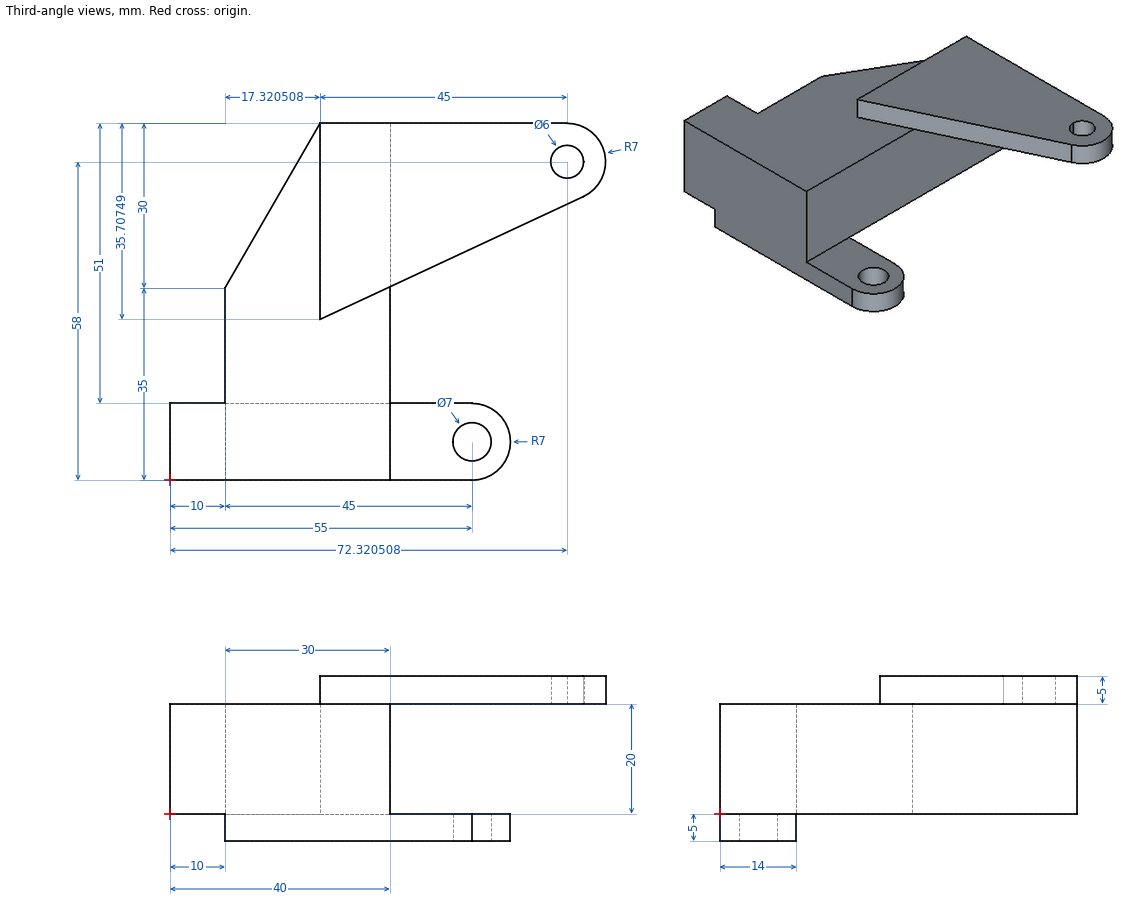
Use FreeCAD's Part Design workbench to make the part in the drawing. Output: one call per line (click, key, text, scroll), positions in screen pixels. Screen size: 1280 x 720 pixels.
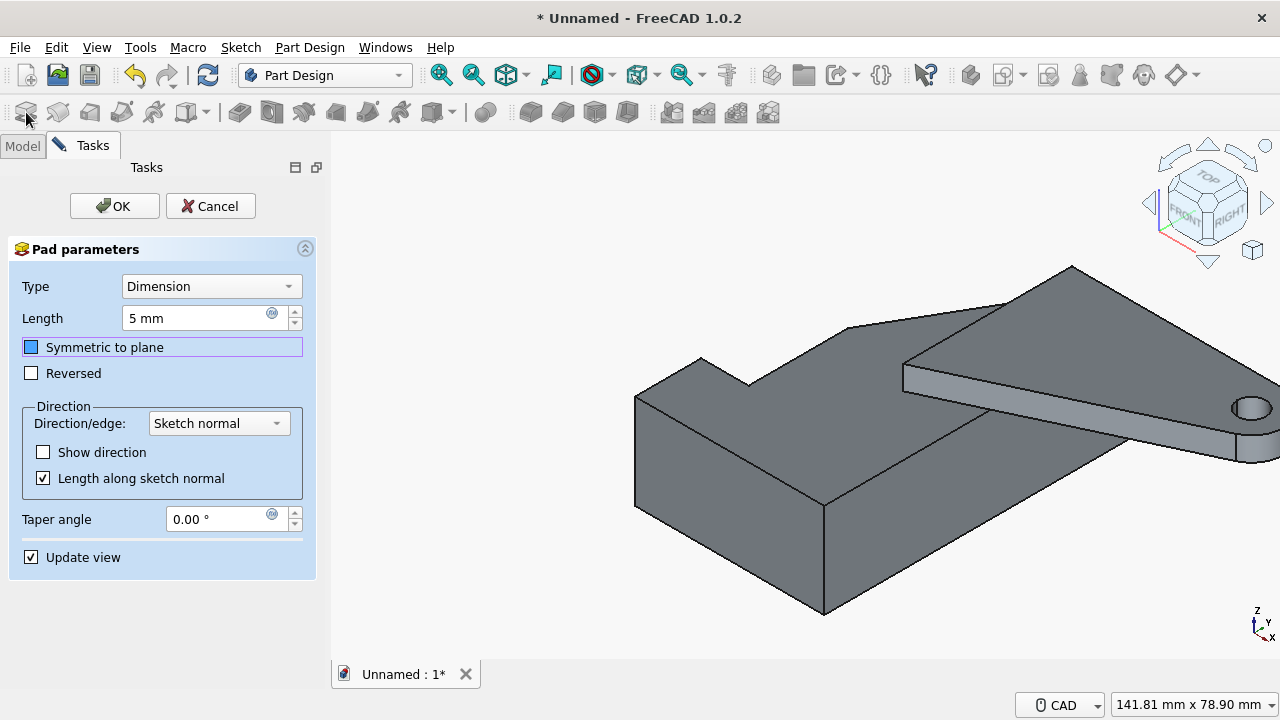
click(115, 206)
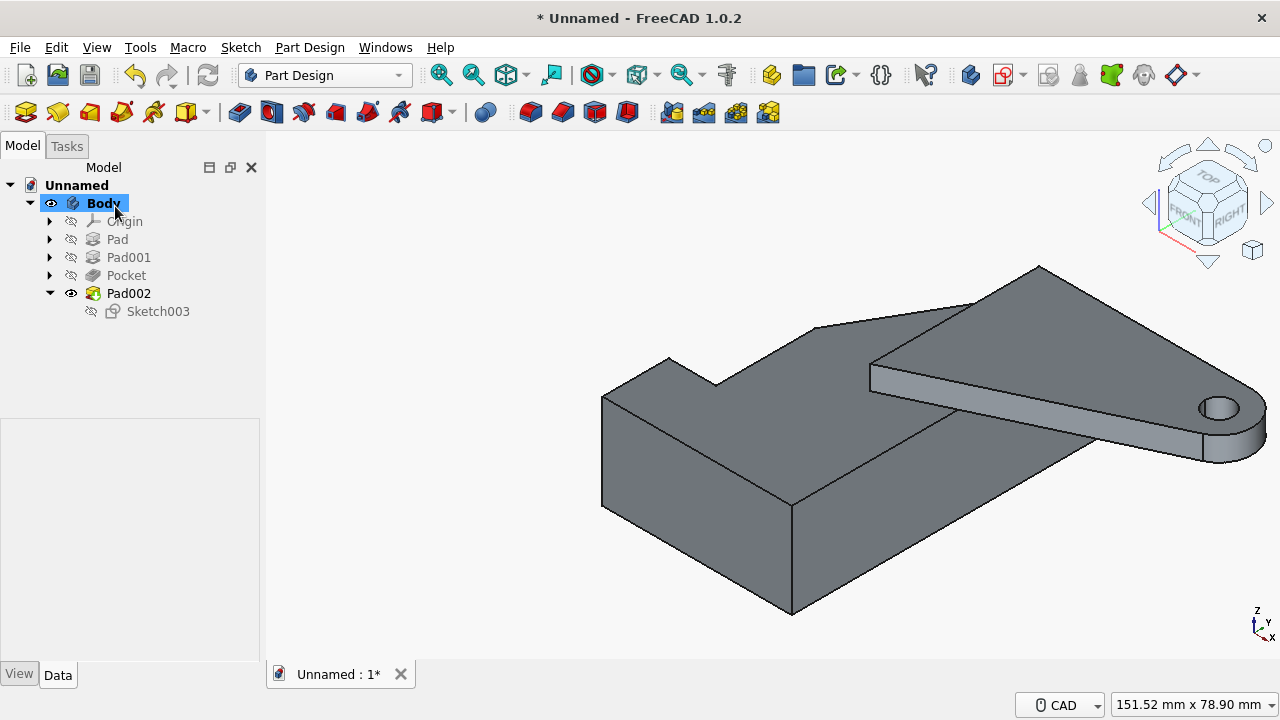
click(442, 76)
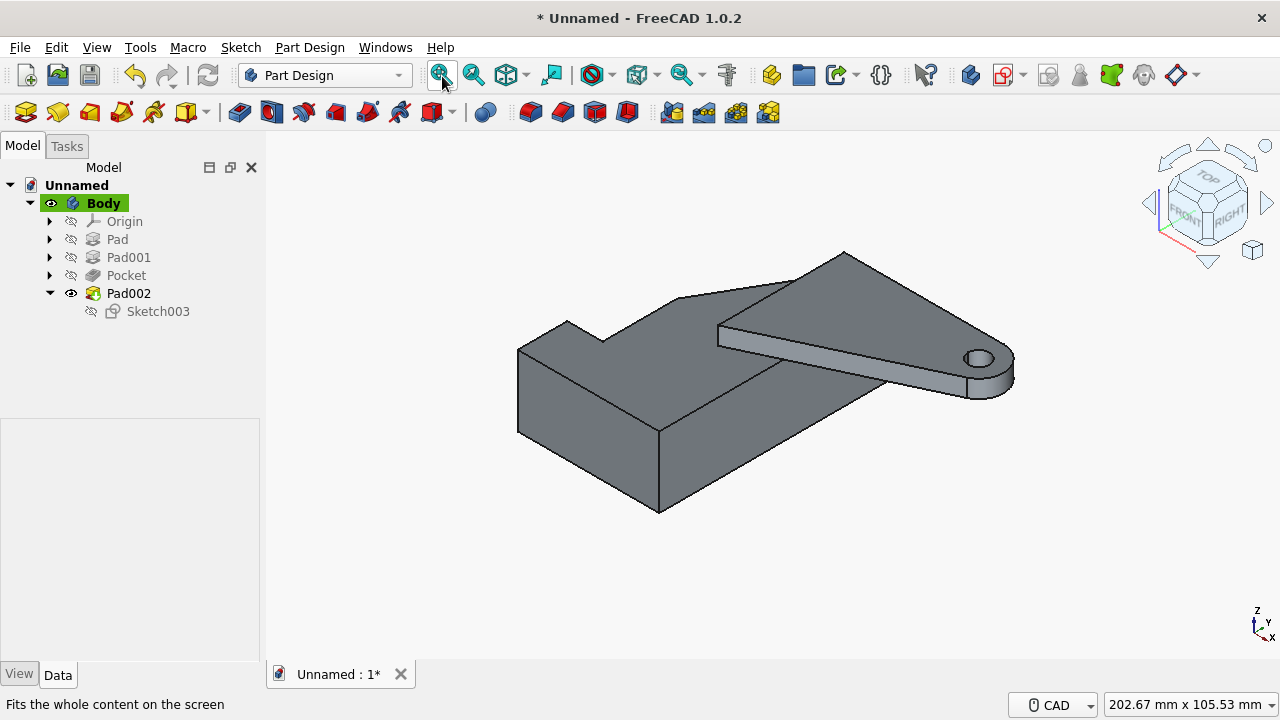
click(1004, 76)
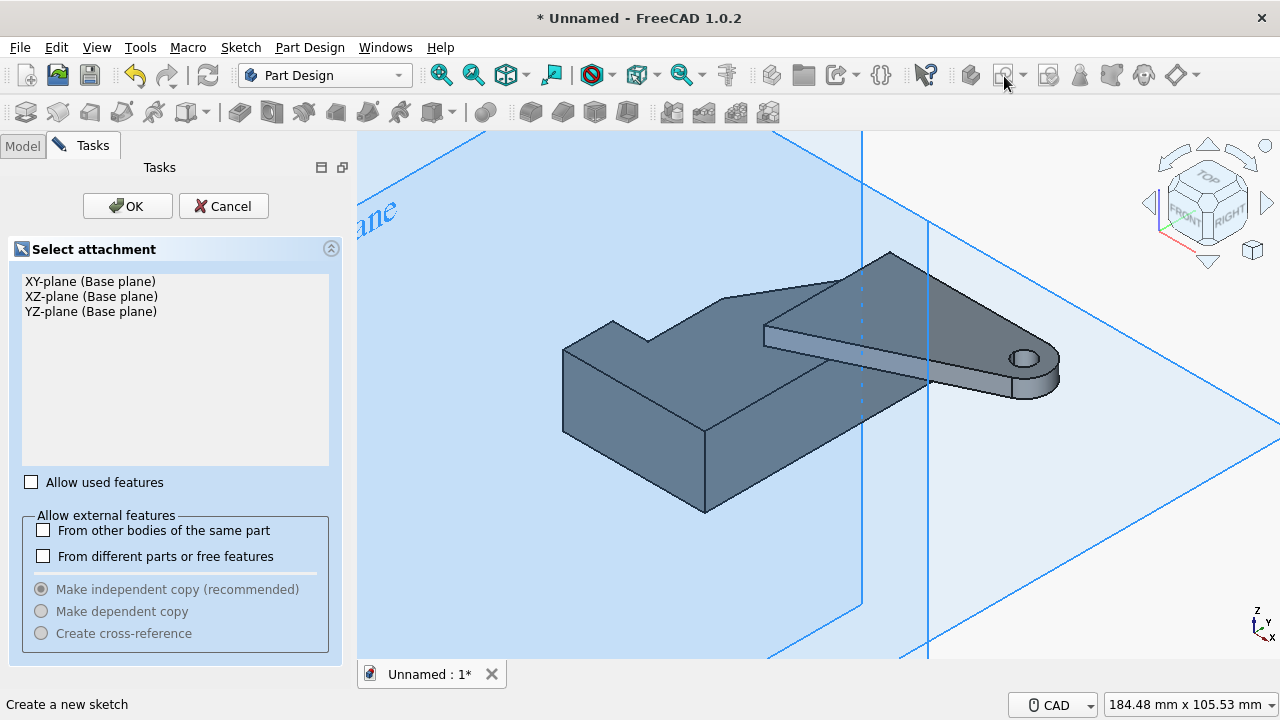
click(82, 282)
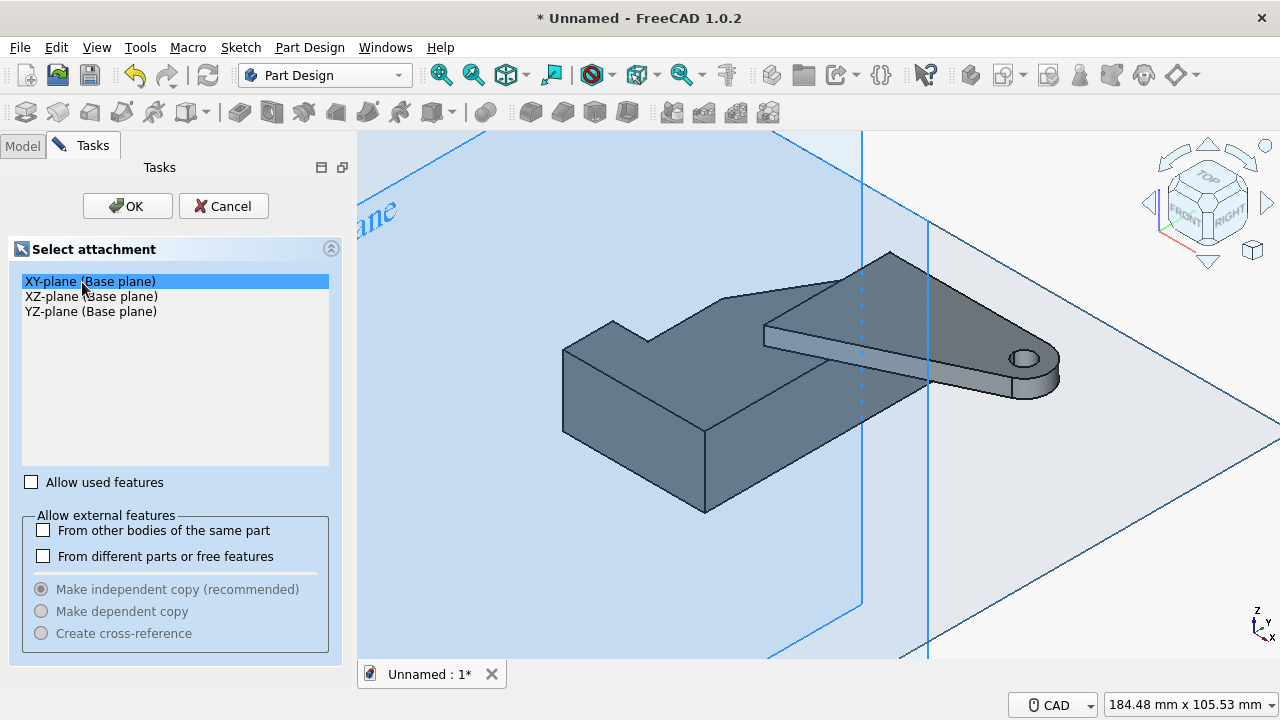
click(128, 206)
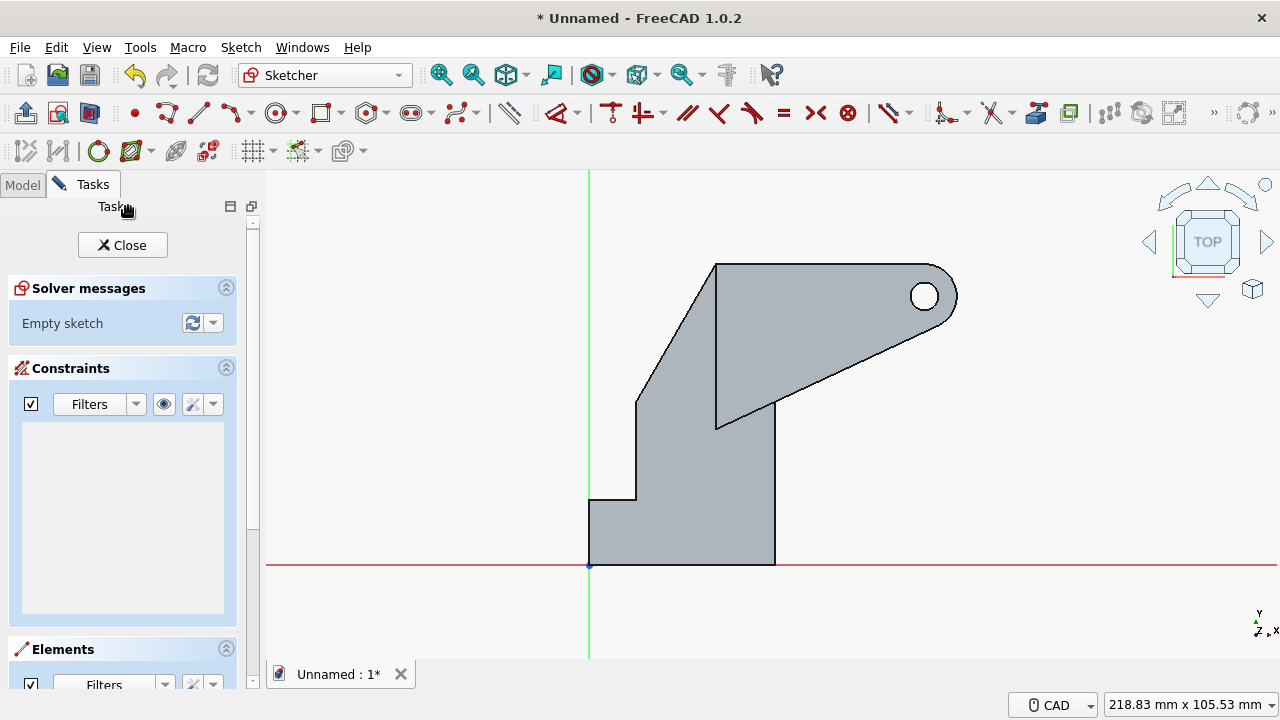
click(90, 114)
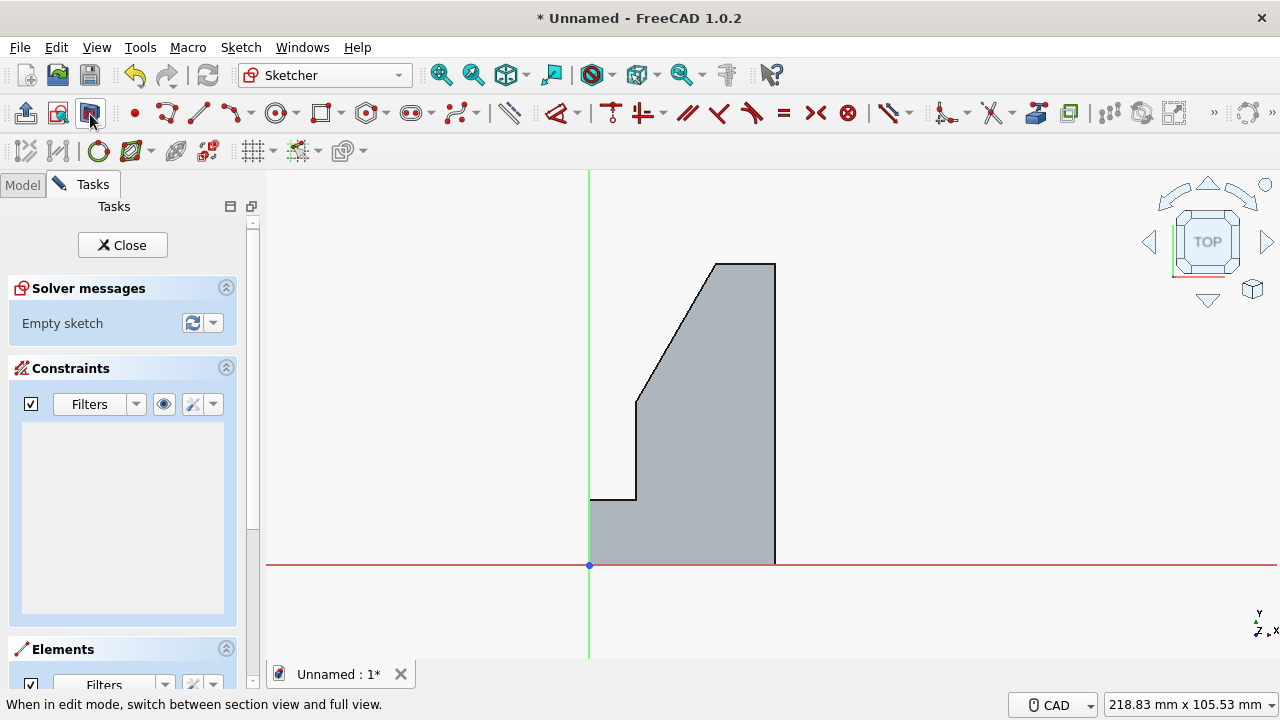
scroll(756, 629, up, 4)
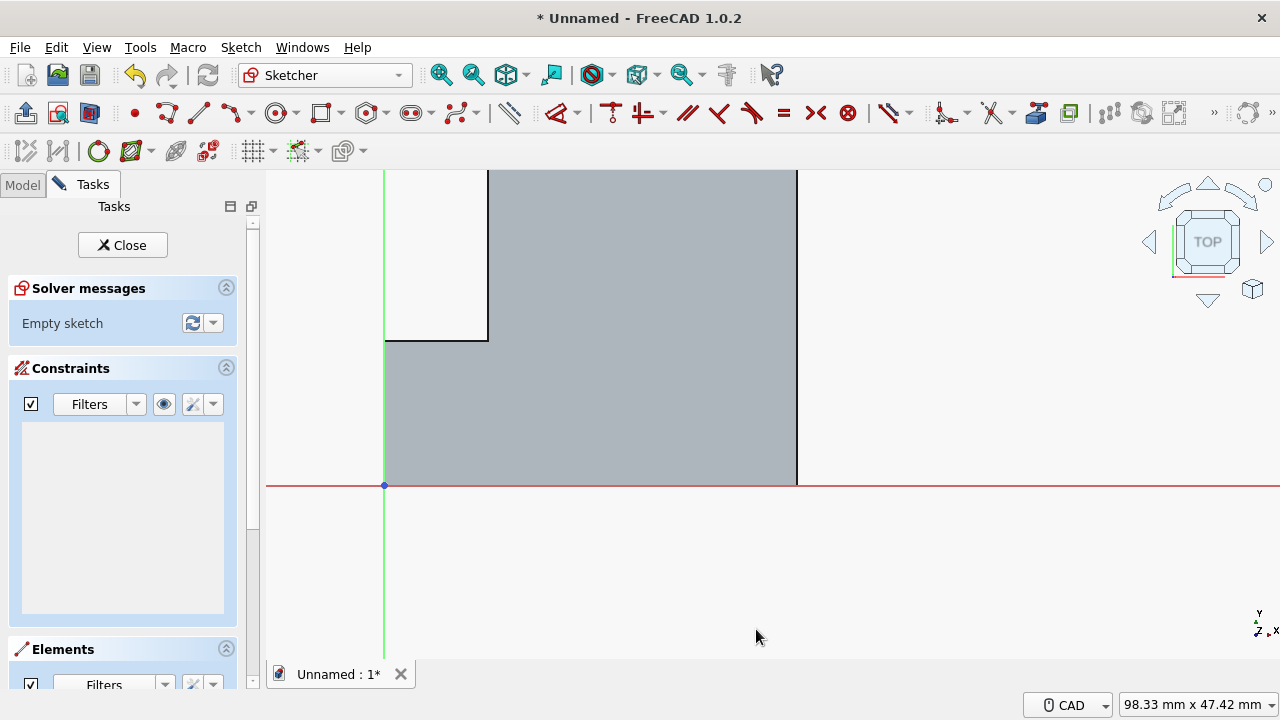
click(168, 114)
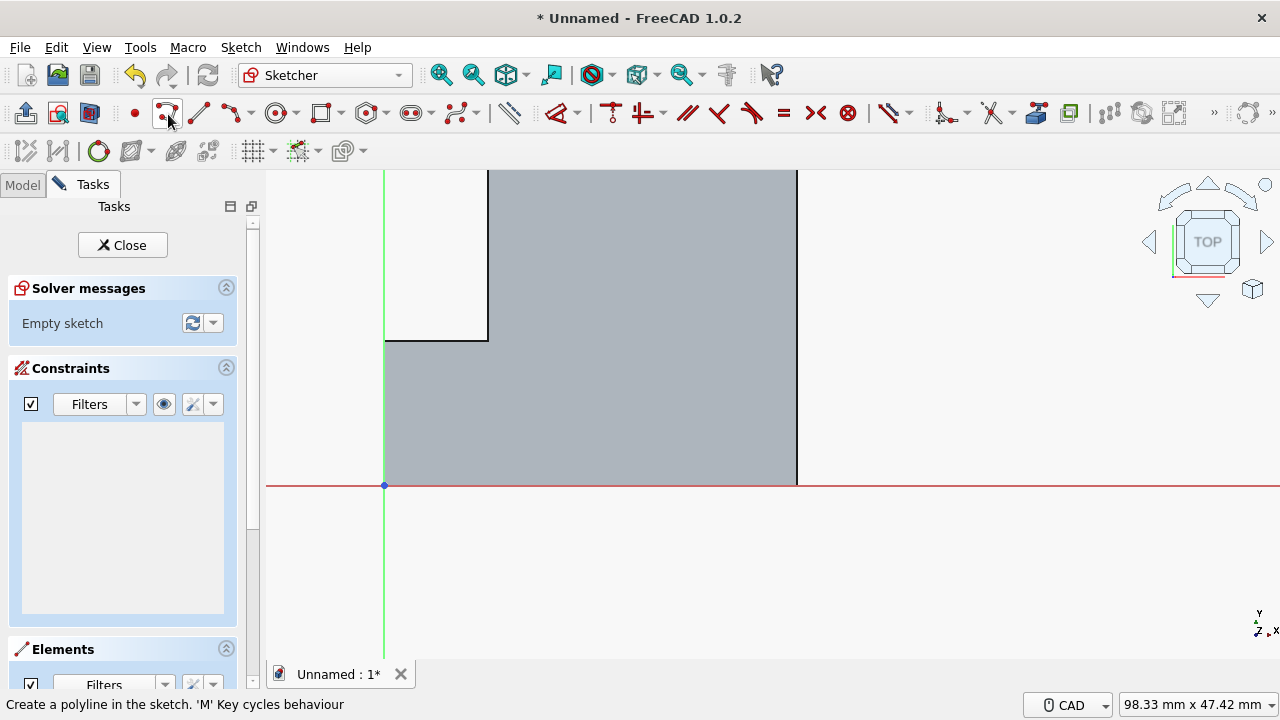
click(952, 486)
click(488, 477)
click(488, 341)
click(952, 341)
right_click(952, 341)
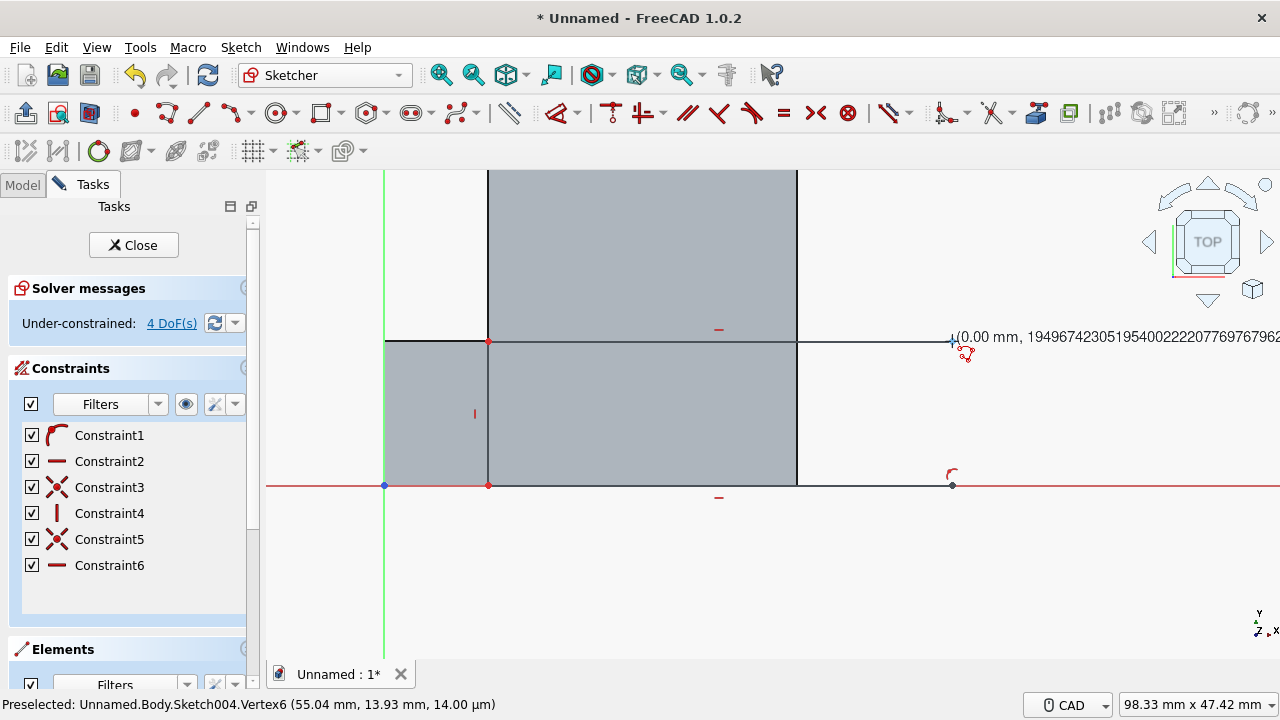
click(232, 114)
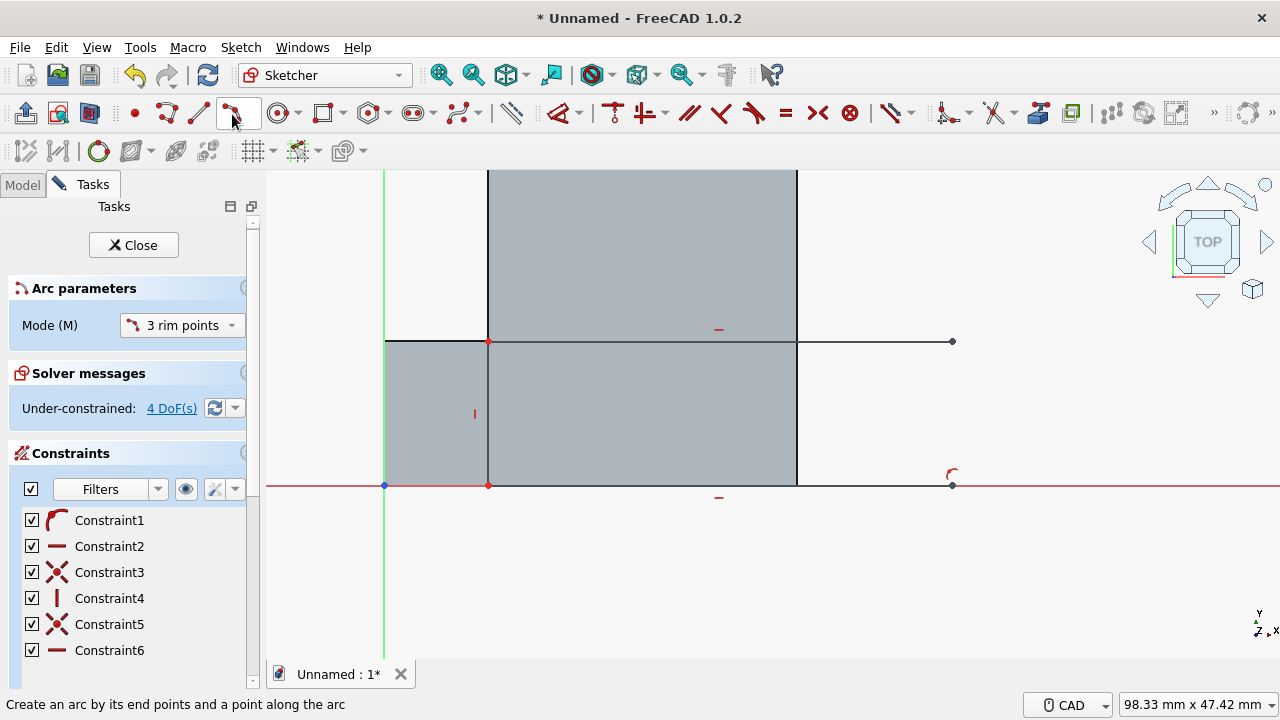
click(952, 342)
click(952, 486)
click(1024, 413)